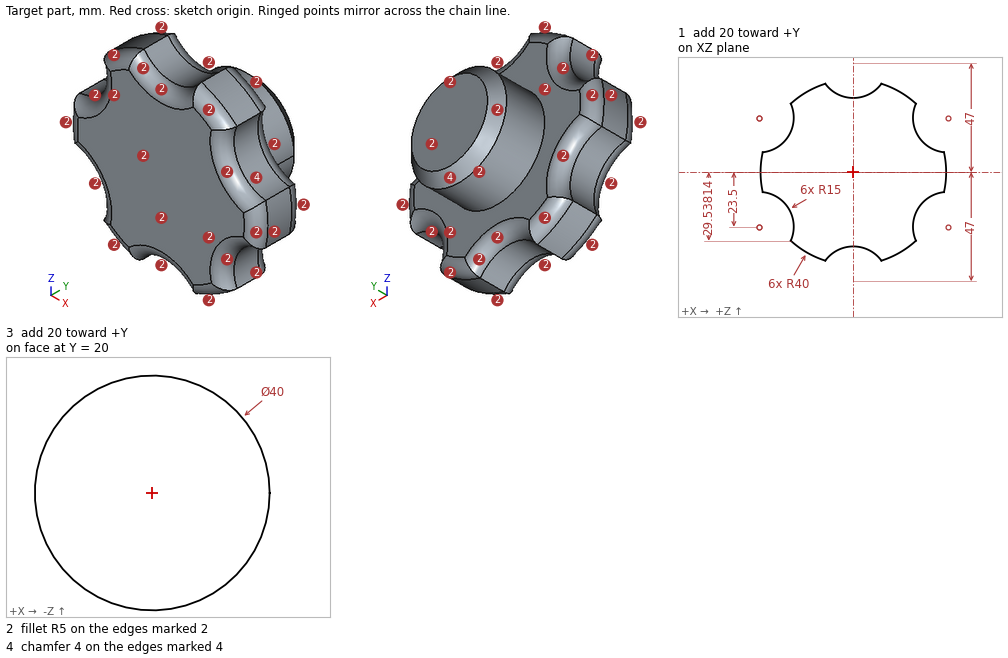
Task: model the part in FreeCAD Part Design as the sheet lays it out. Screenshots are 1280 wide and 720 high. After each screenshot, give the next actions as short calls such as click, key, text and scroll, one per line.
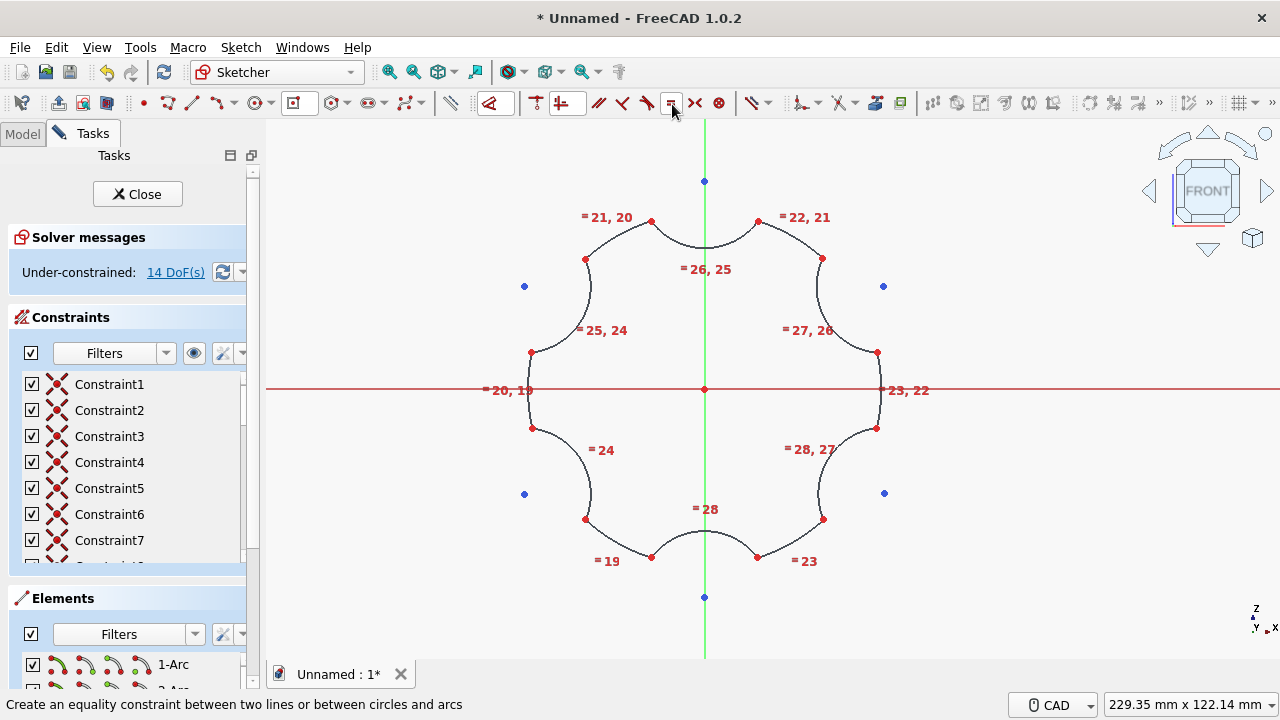
click(705, 182)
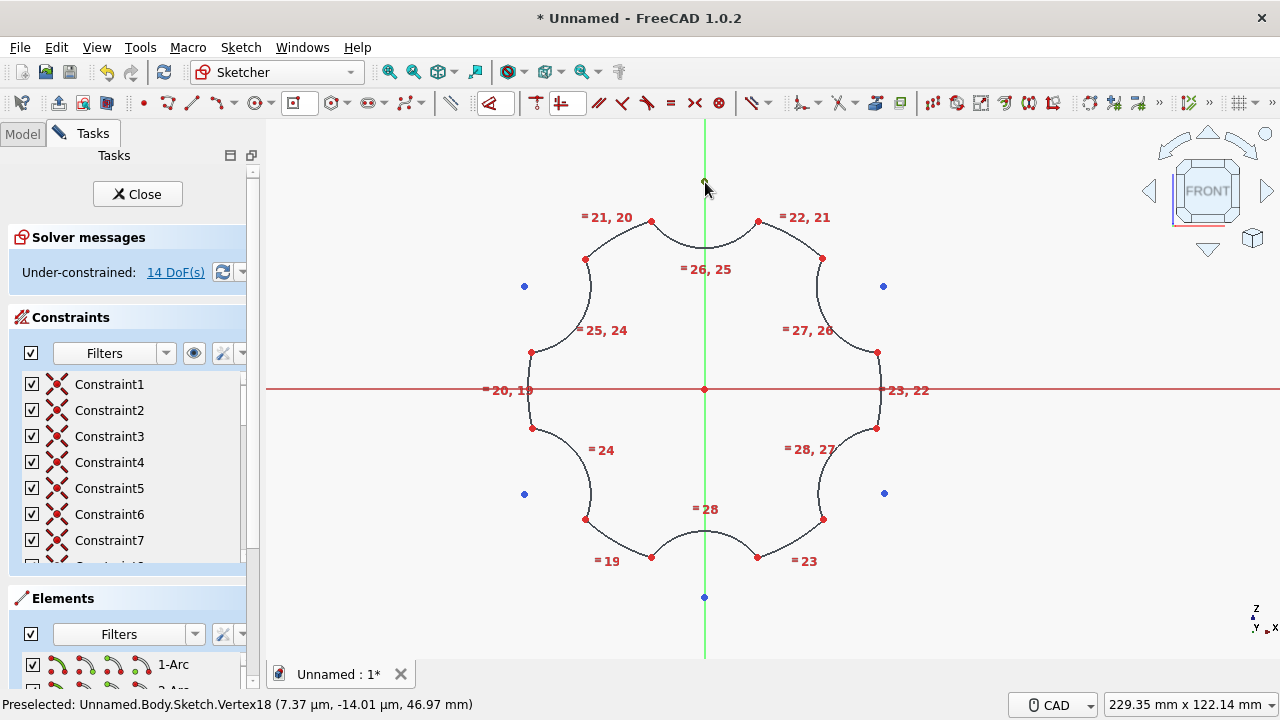
click(705, 562)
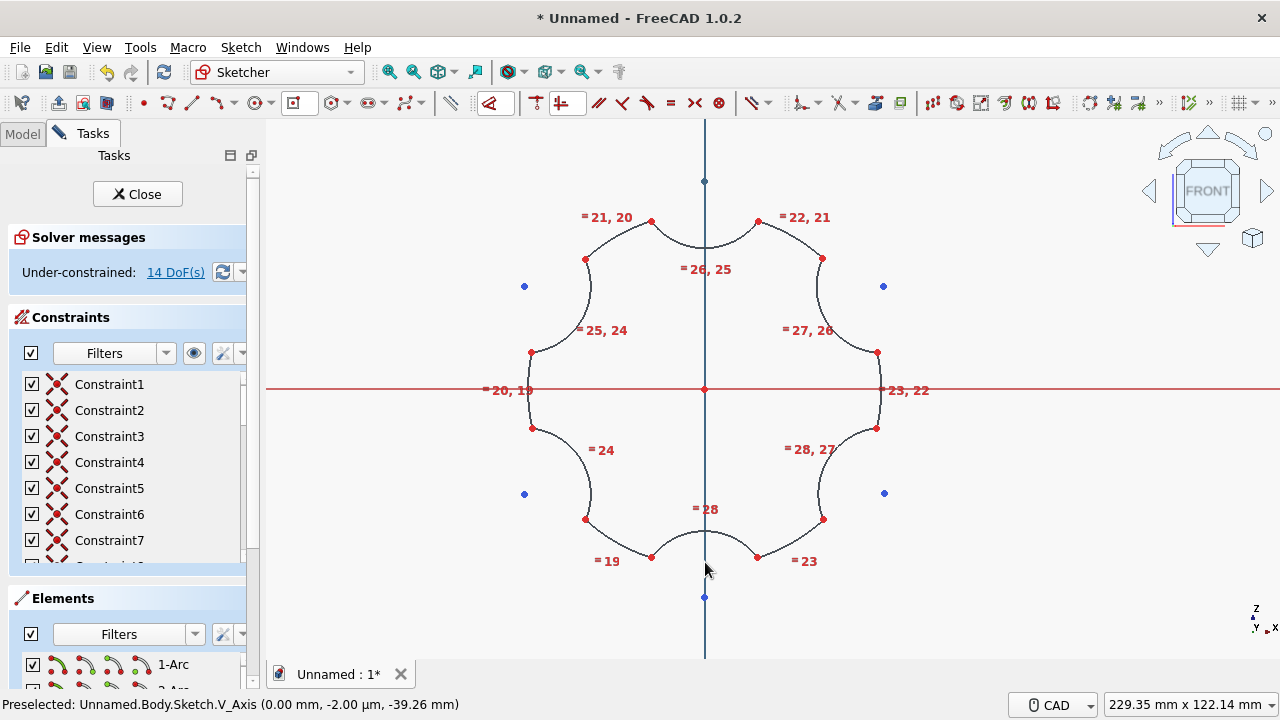
click(536, 104)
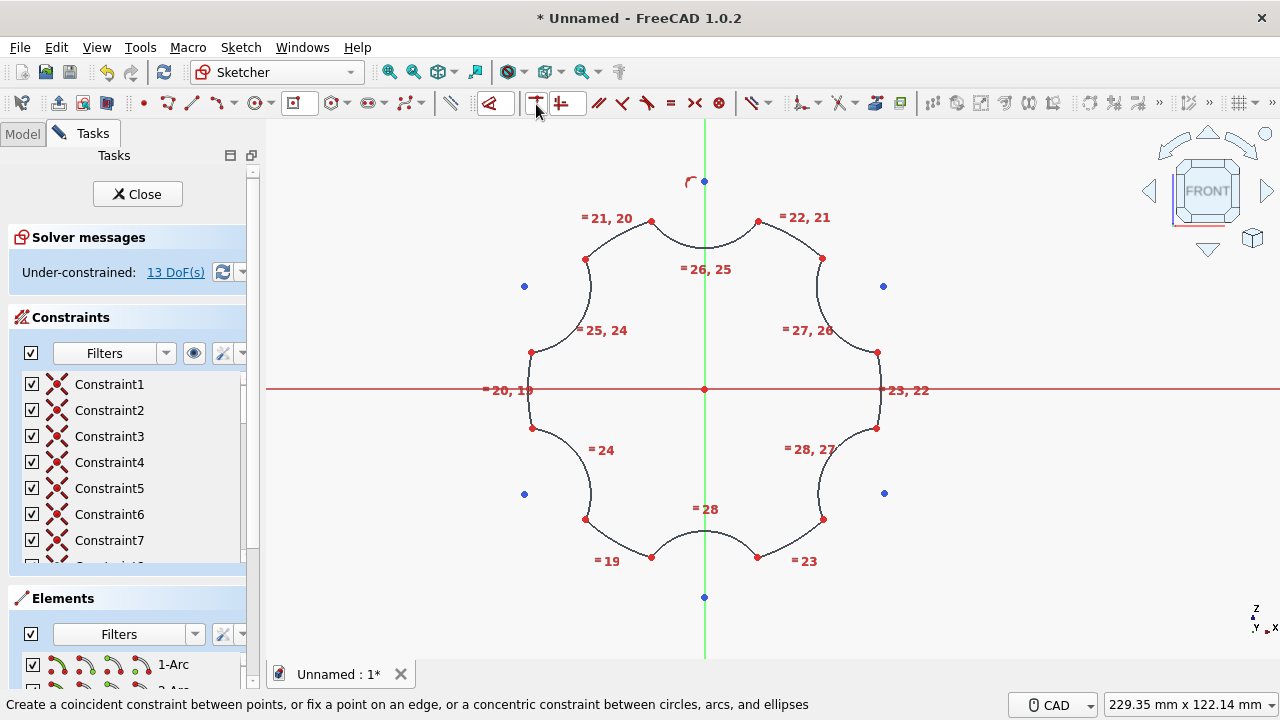
click(704, 598)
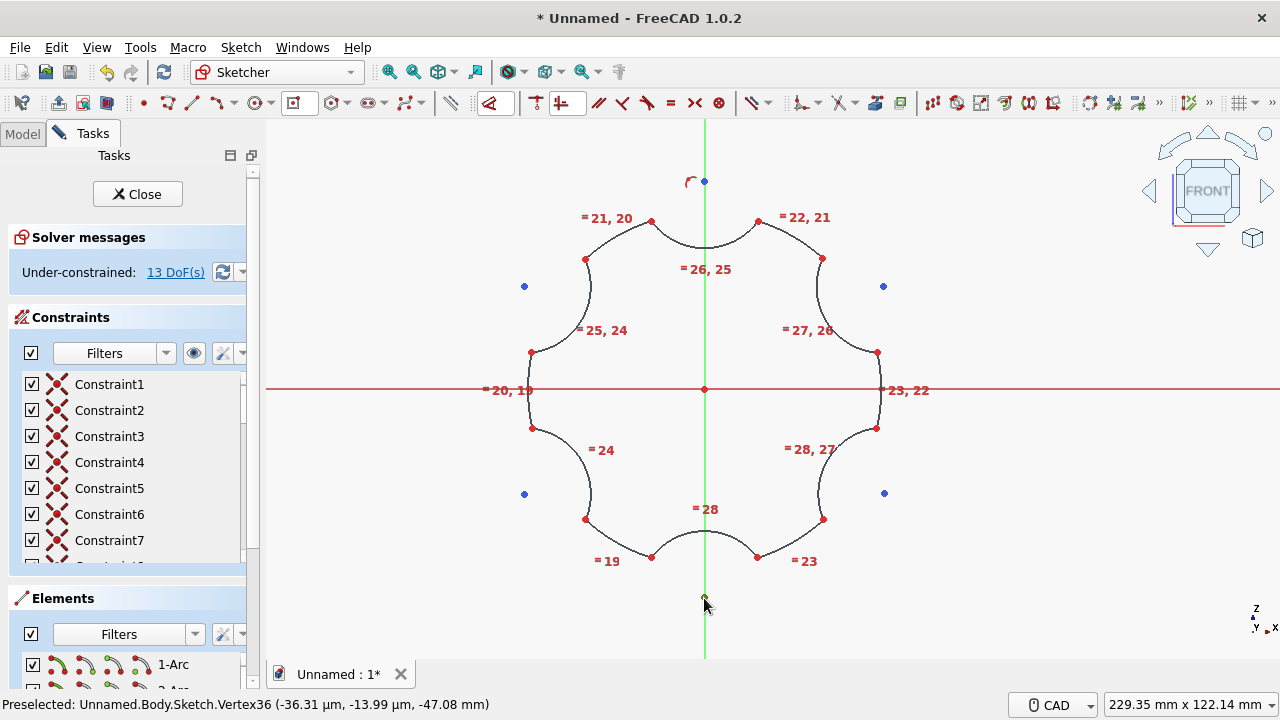
click(705, 562)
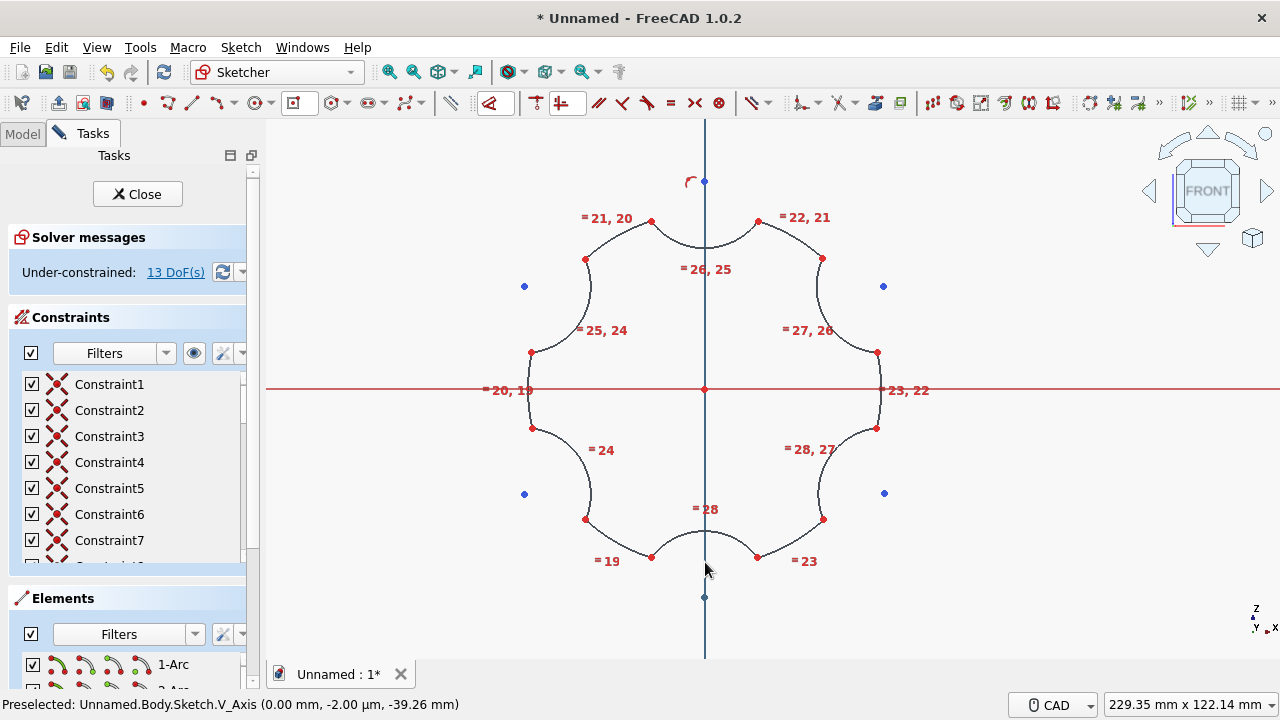
click(536, 104)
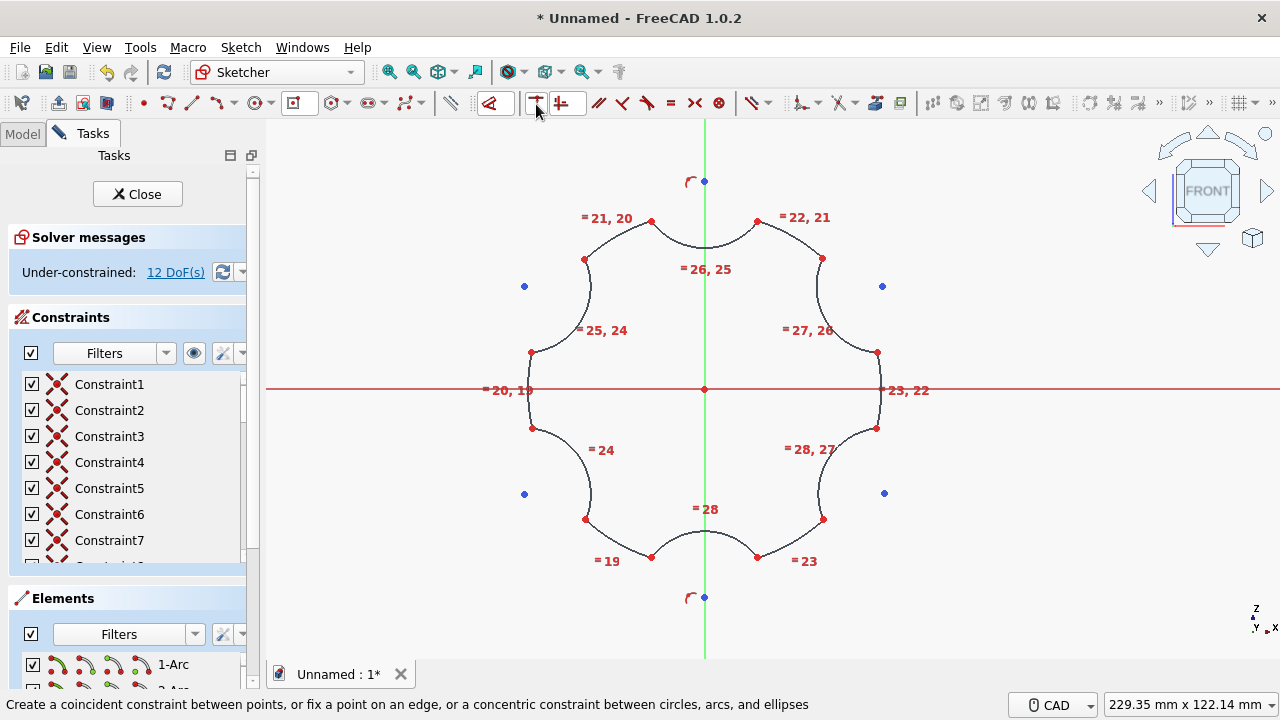
click(525, 494)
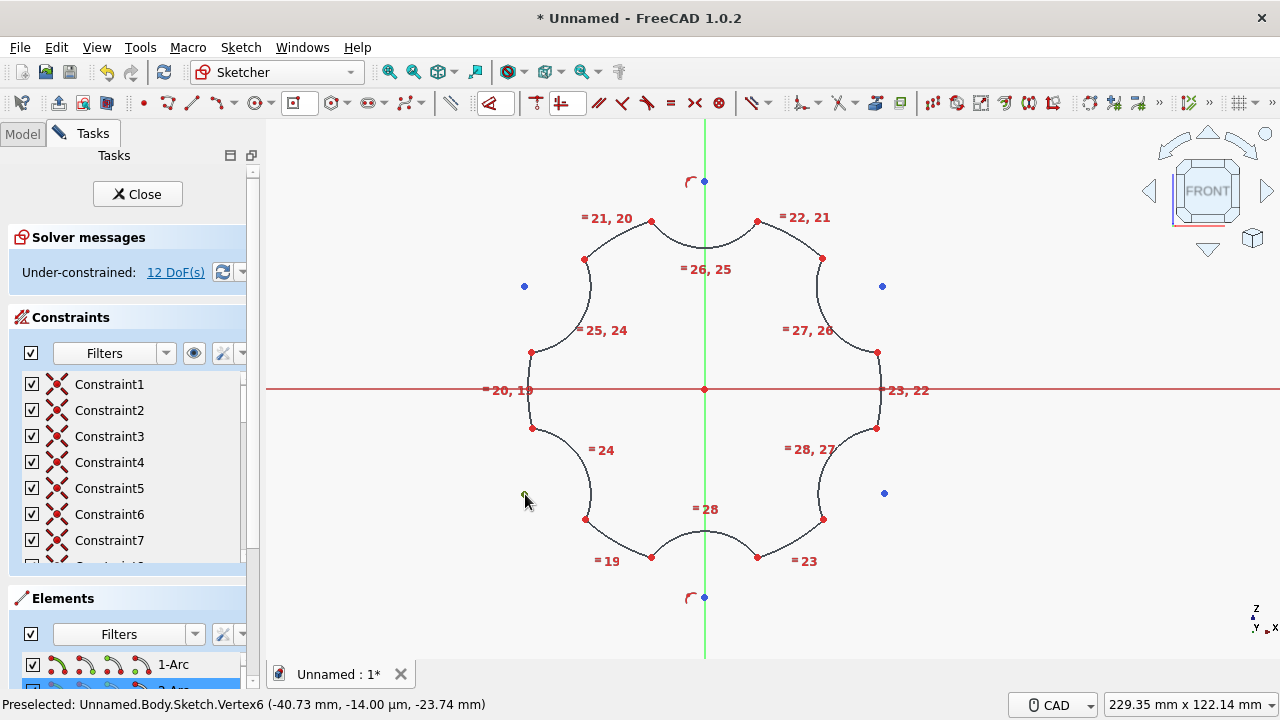
click(524, 287)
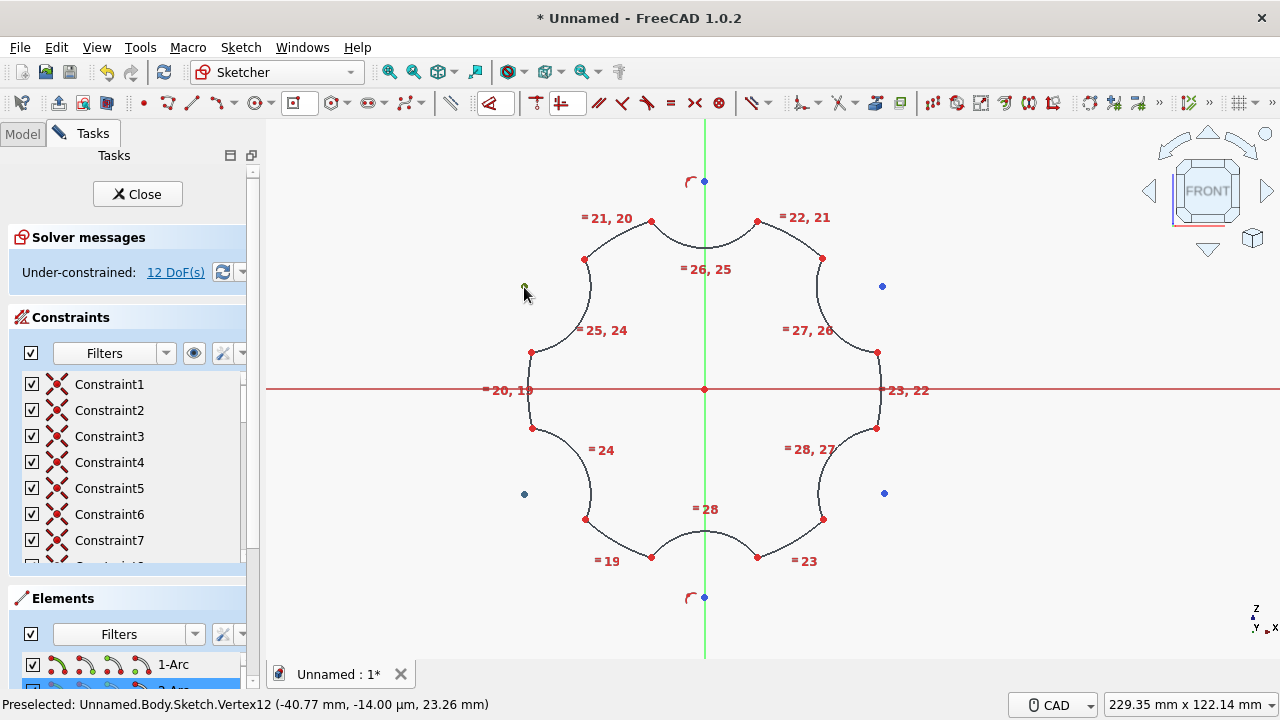
click(353, 389)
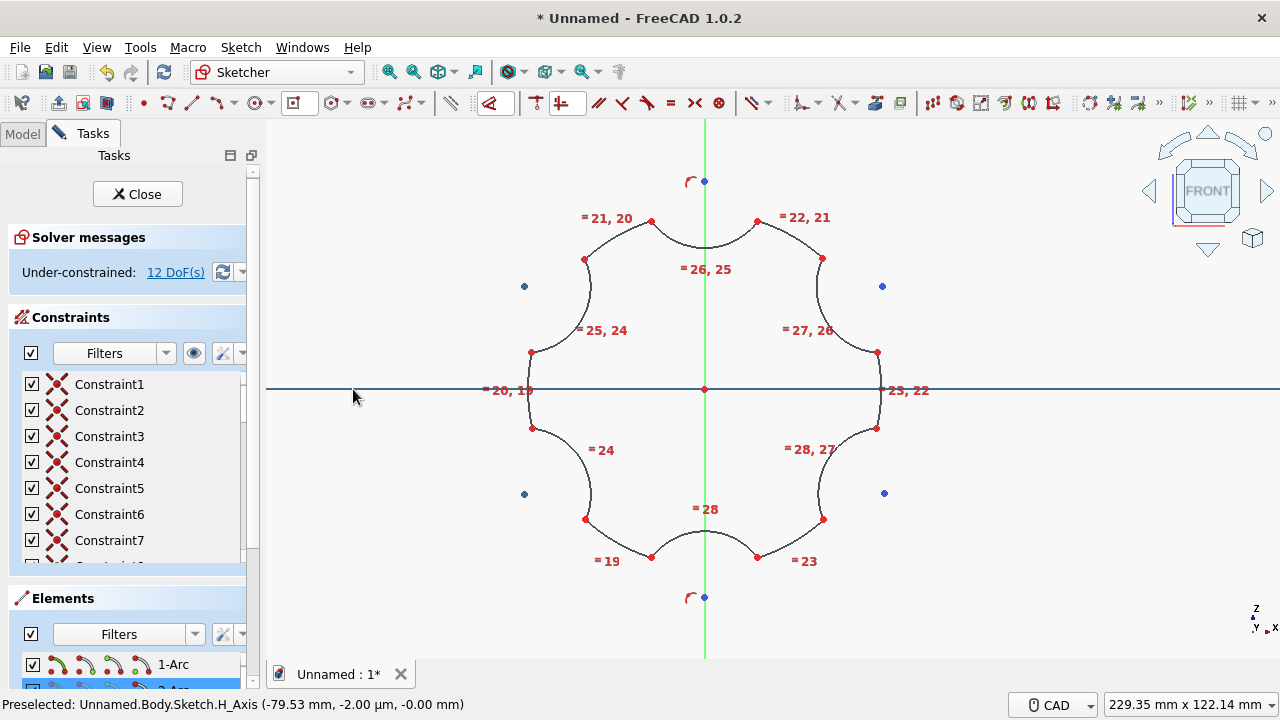
click(696, 104)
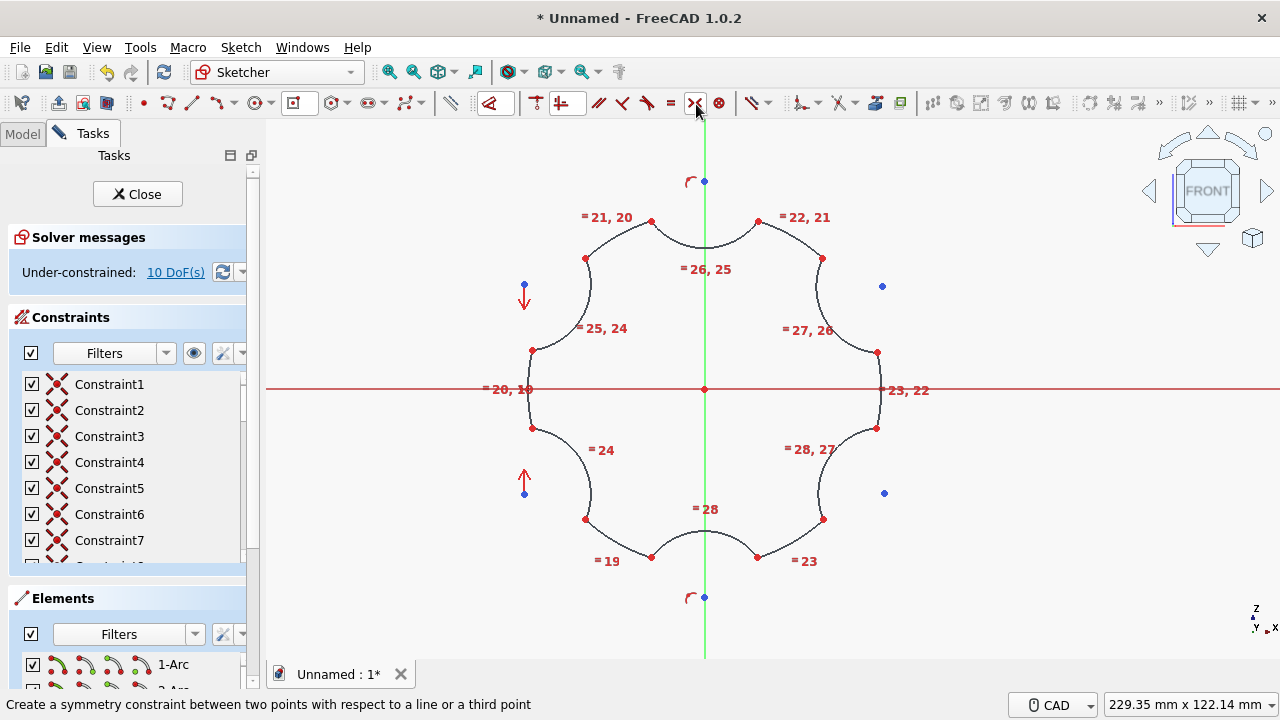
click(524, 284)